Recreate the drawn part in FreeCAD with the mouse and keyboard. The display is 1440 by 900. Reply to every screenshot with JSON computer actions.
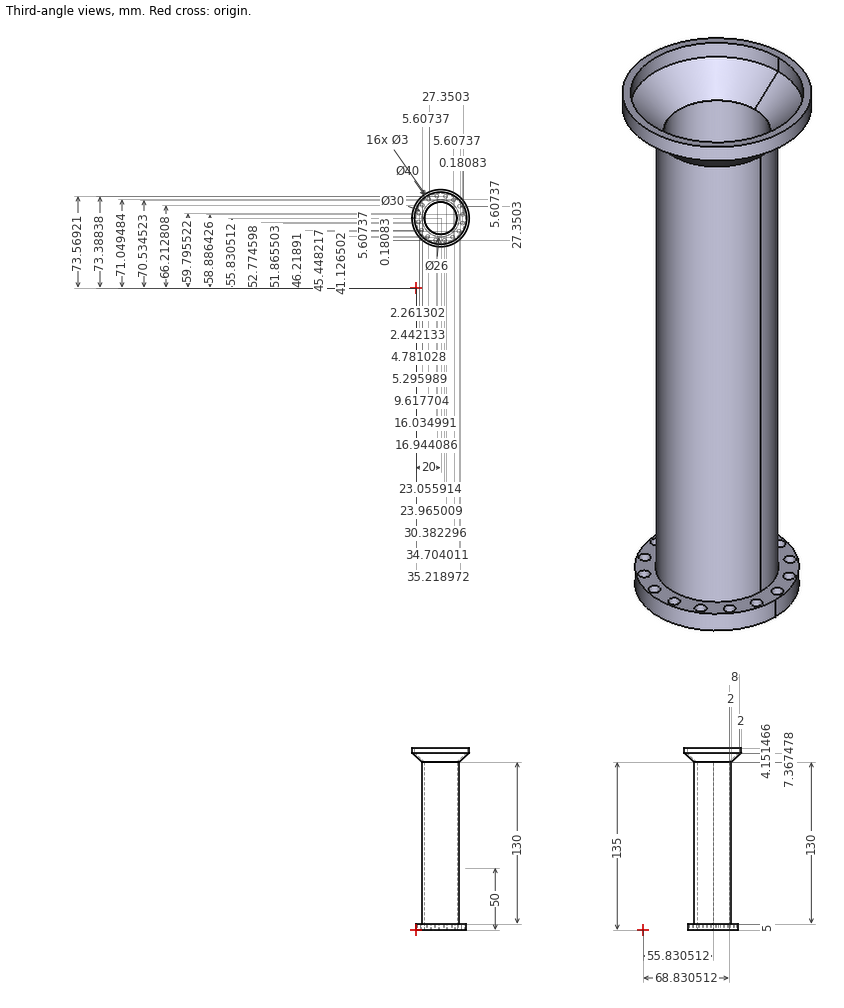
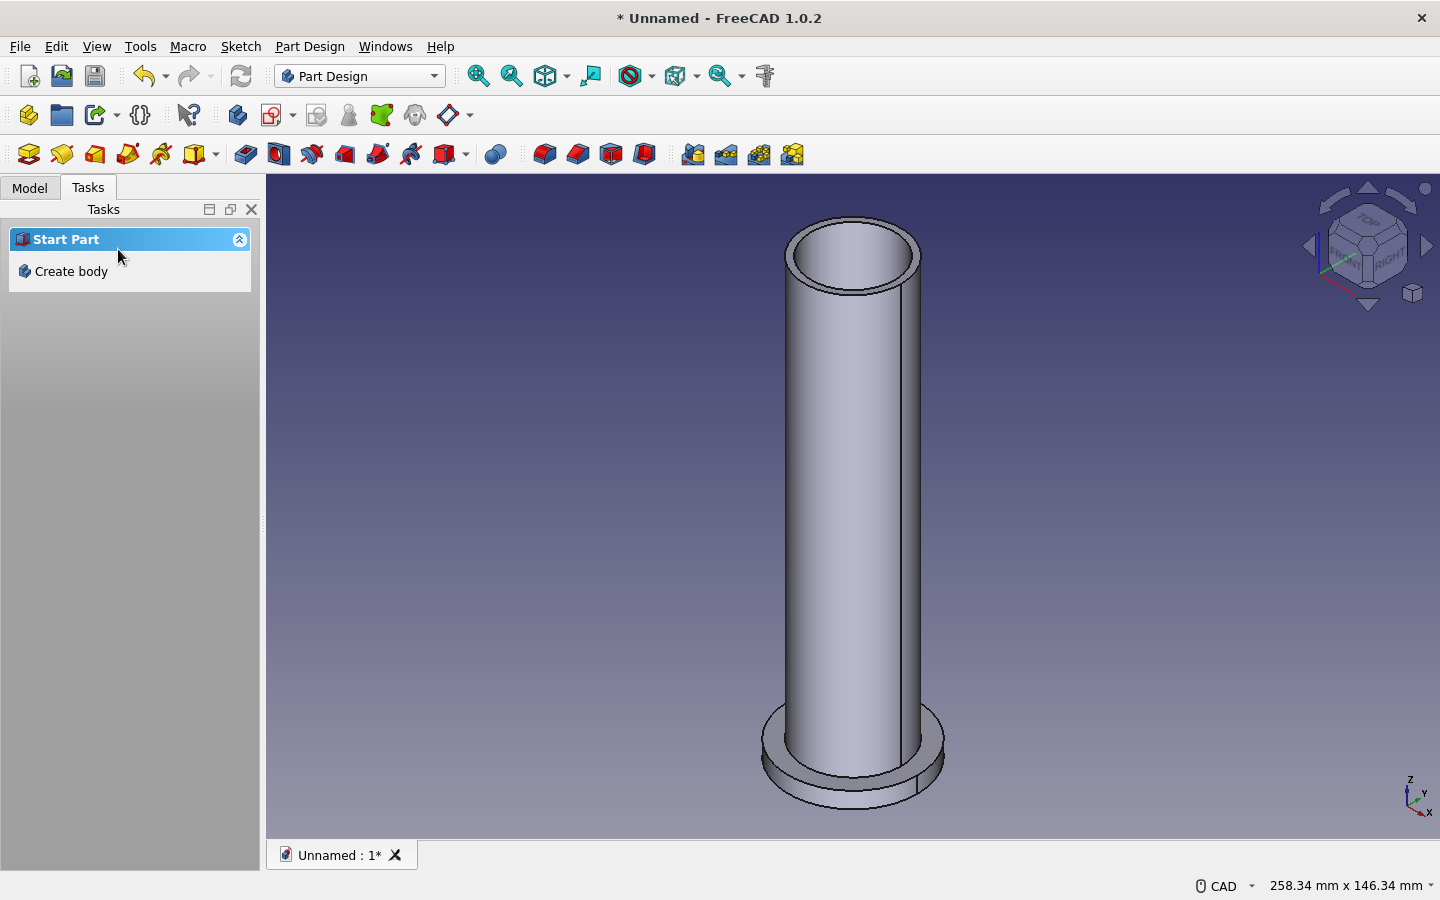
{"action": "left_click", "coordinate": [270, 116]}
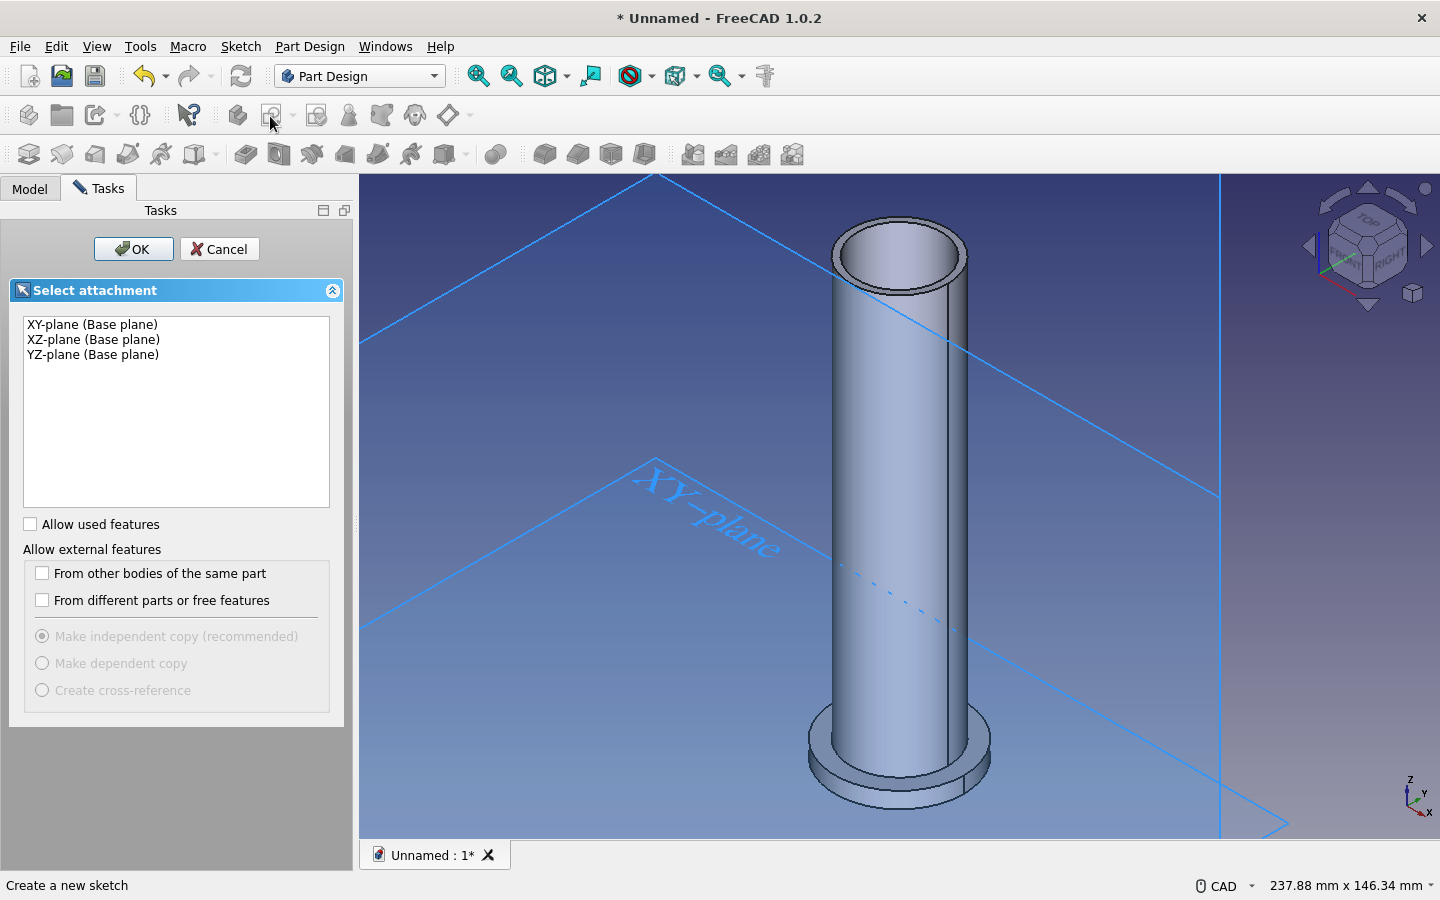
{"action": "left_click", "coordinate": [84, 324]}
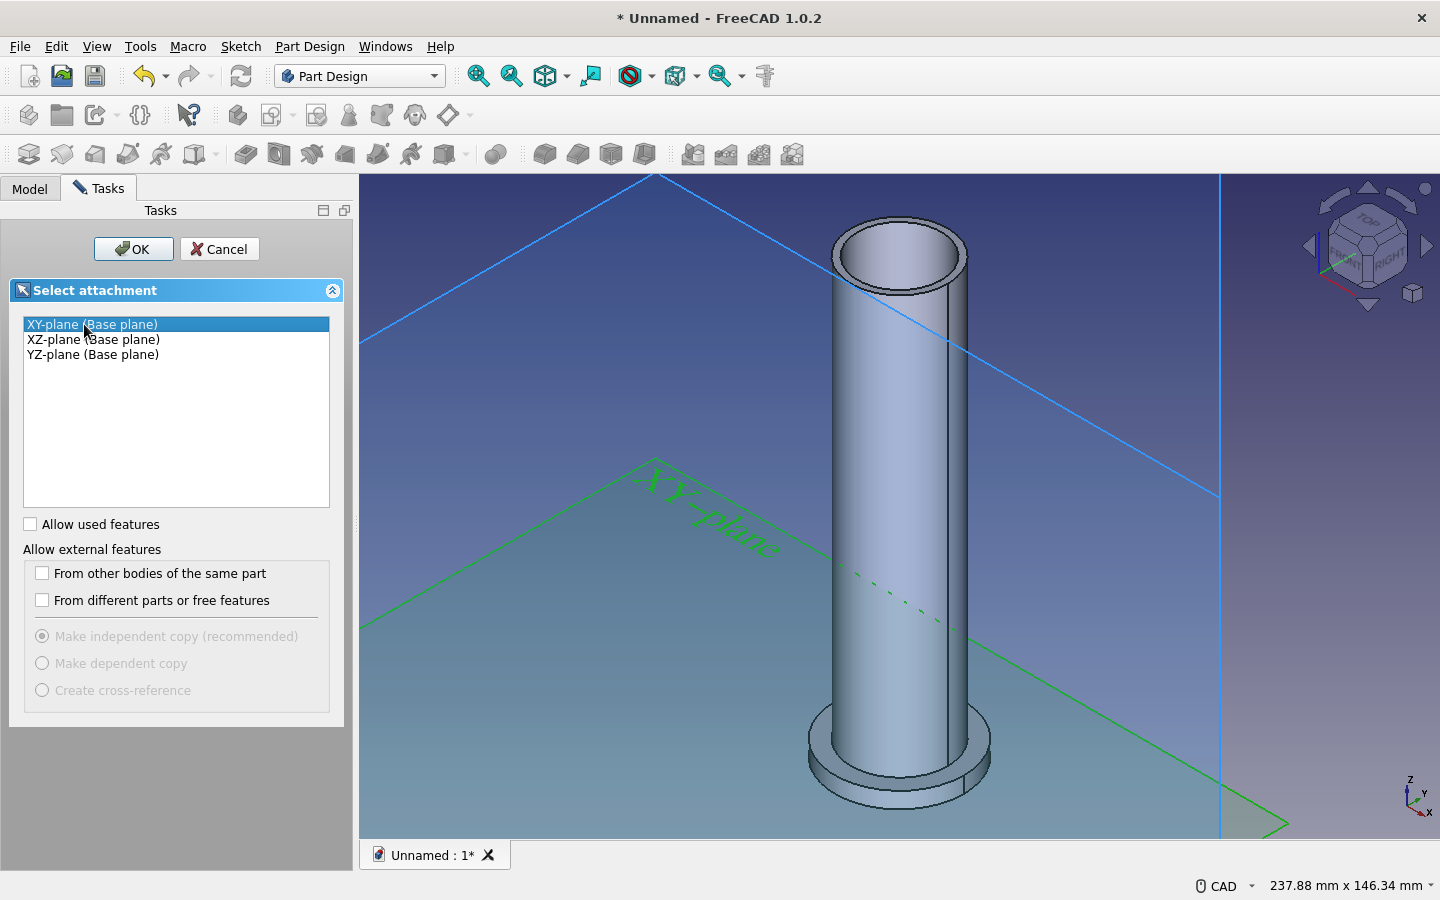
{"action": "left_click", "coordinate": [134, 249]}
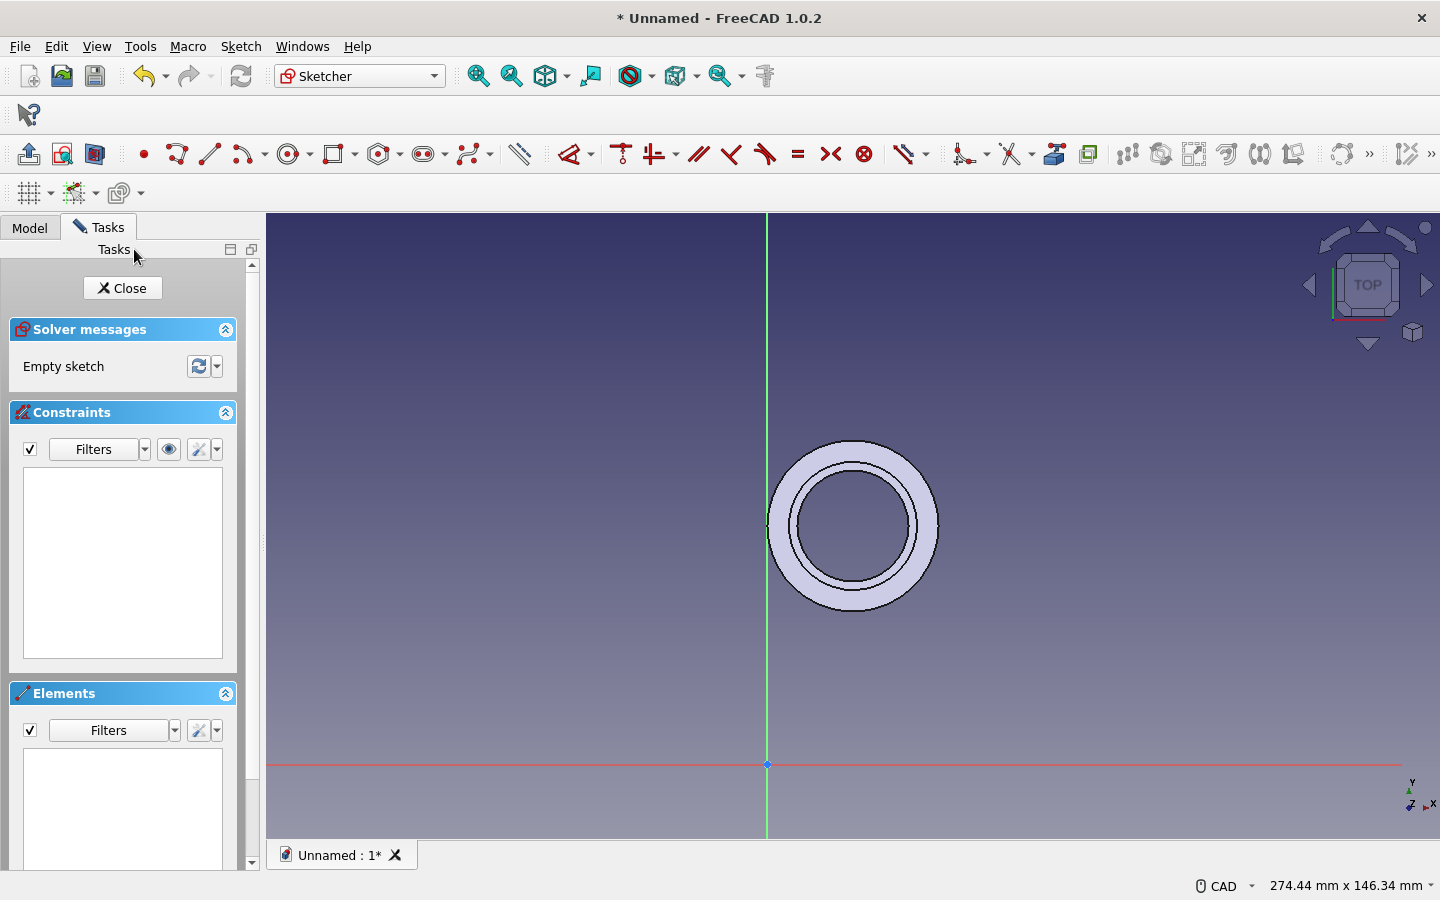
{"action": "left_click", "coordinate": [95, 154]}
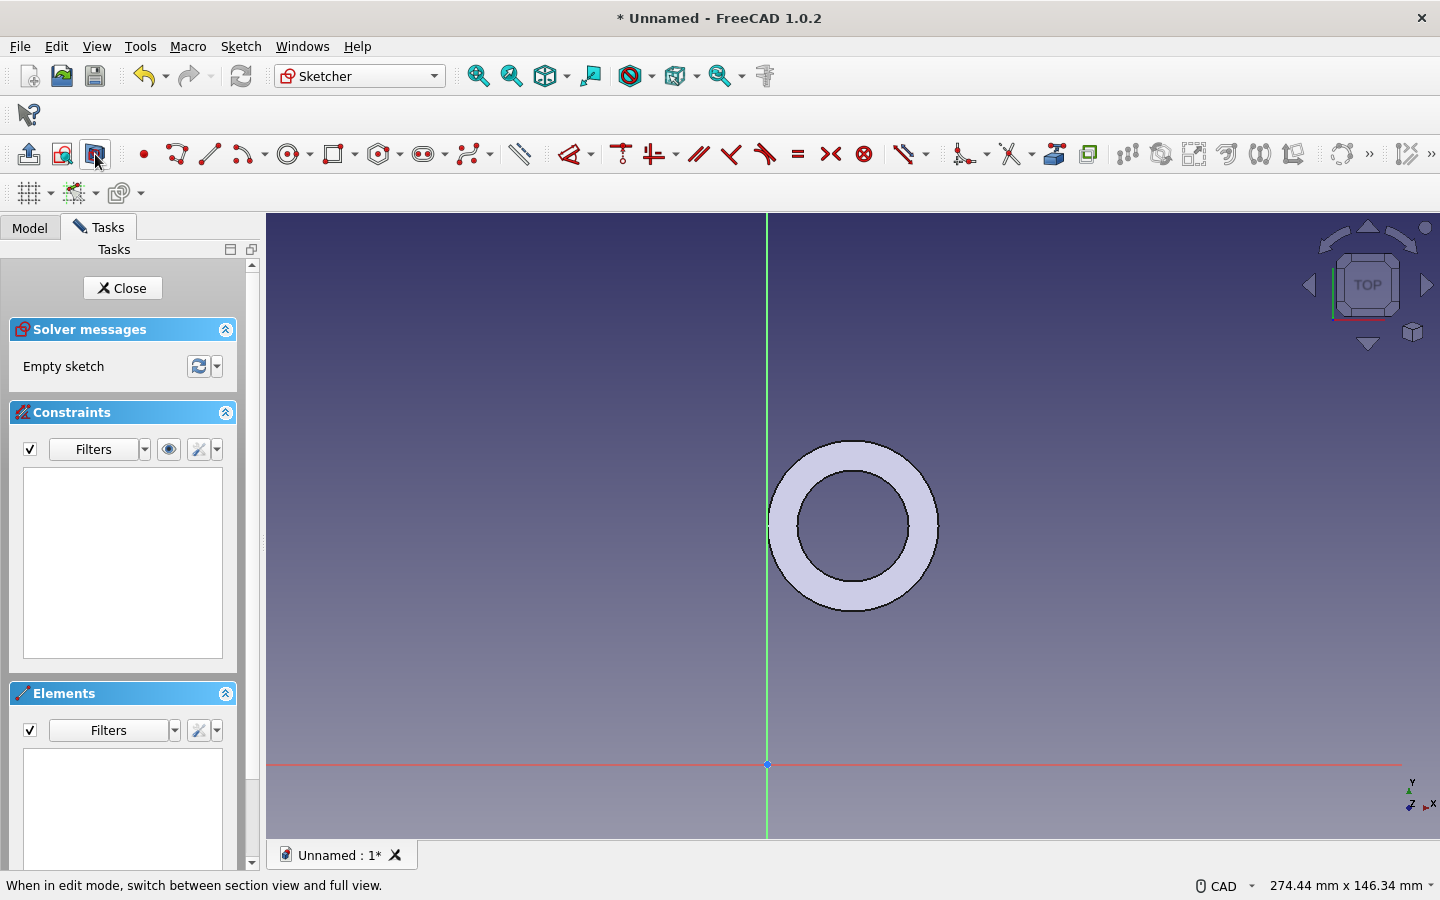
{"action": "left_click", "coordinate": [288, 154]}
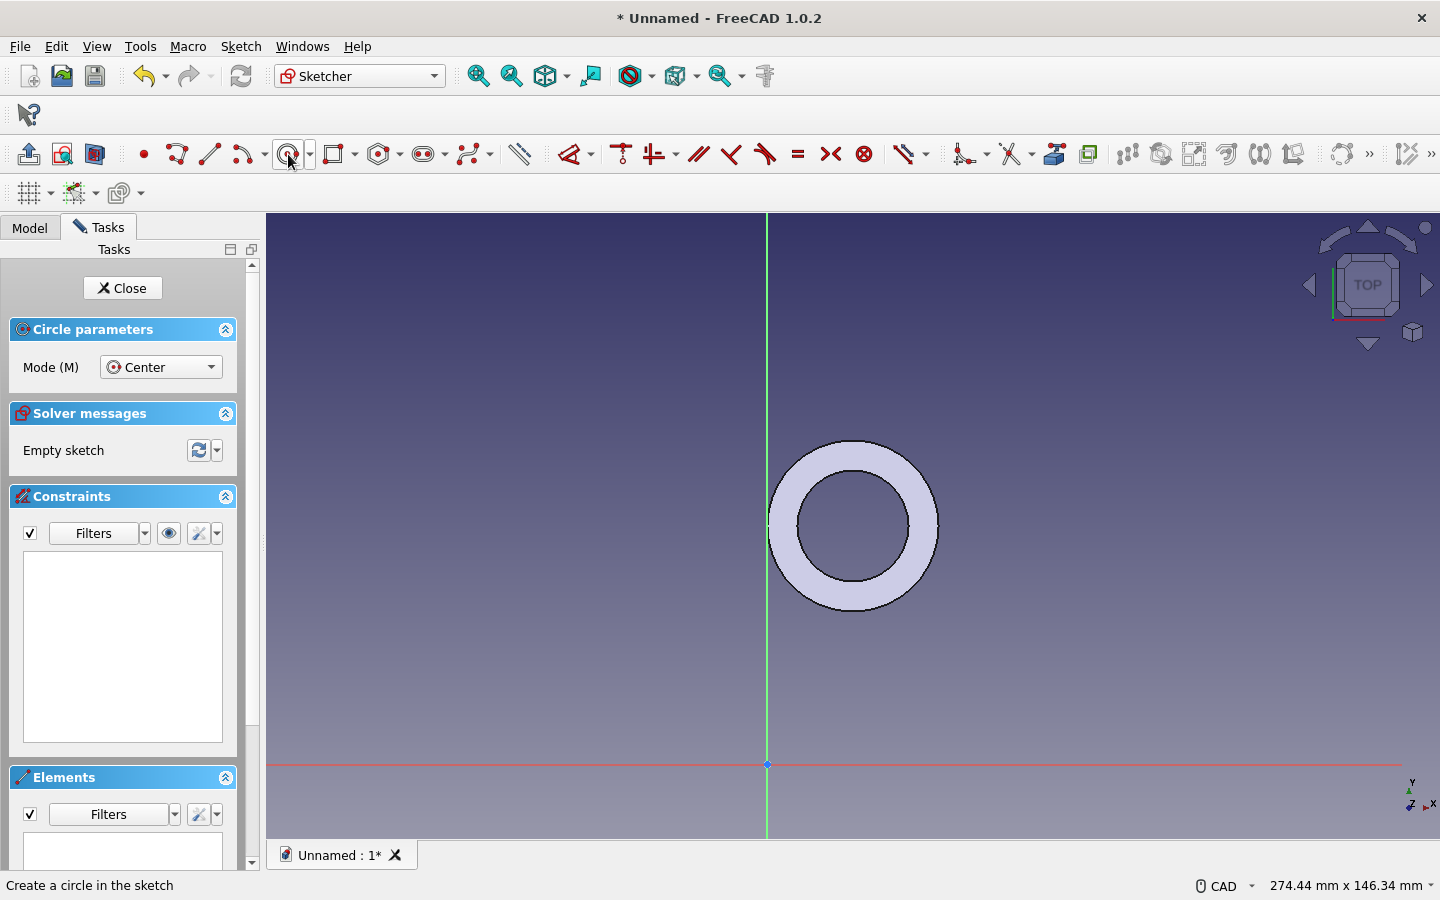
{"action": "scroll", "coordinate": [812, 461], "scroll_direction": "up", "scroll_amount": 7}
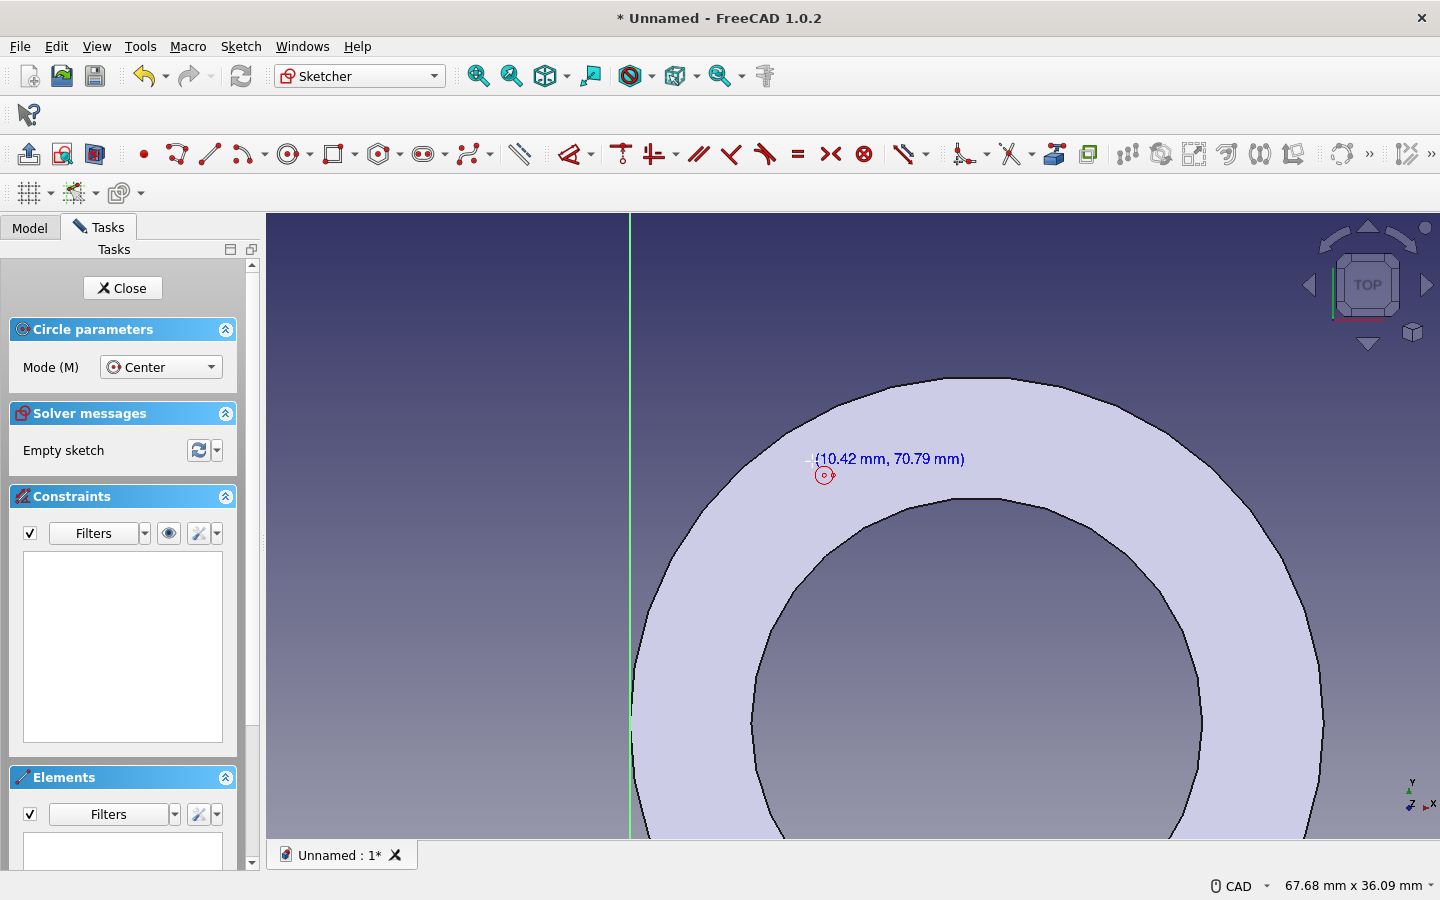
{"action": "scroll", "coordinate": [704, 304], "scroll_direction": "down", "scroll_amount": 6}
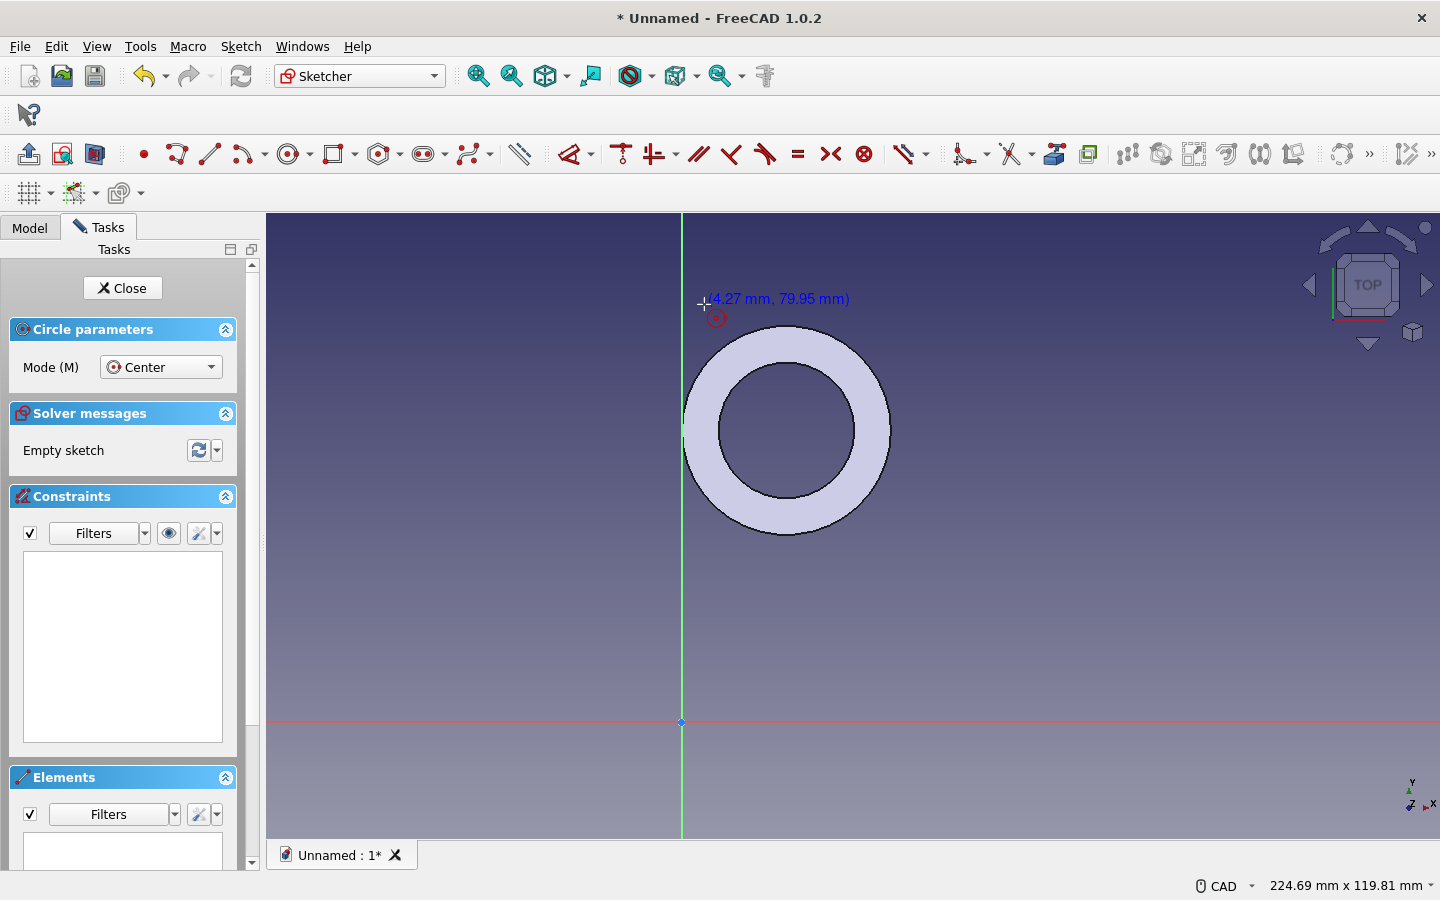
{"action": "left_click", "coordinate": [736, 351]}
{"action": "mouse_move", "coordinate": [742, 345]}